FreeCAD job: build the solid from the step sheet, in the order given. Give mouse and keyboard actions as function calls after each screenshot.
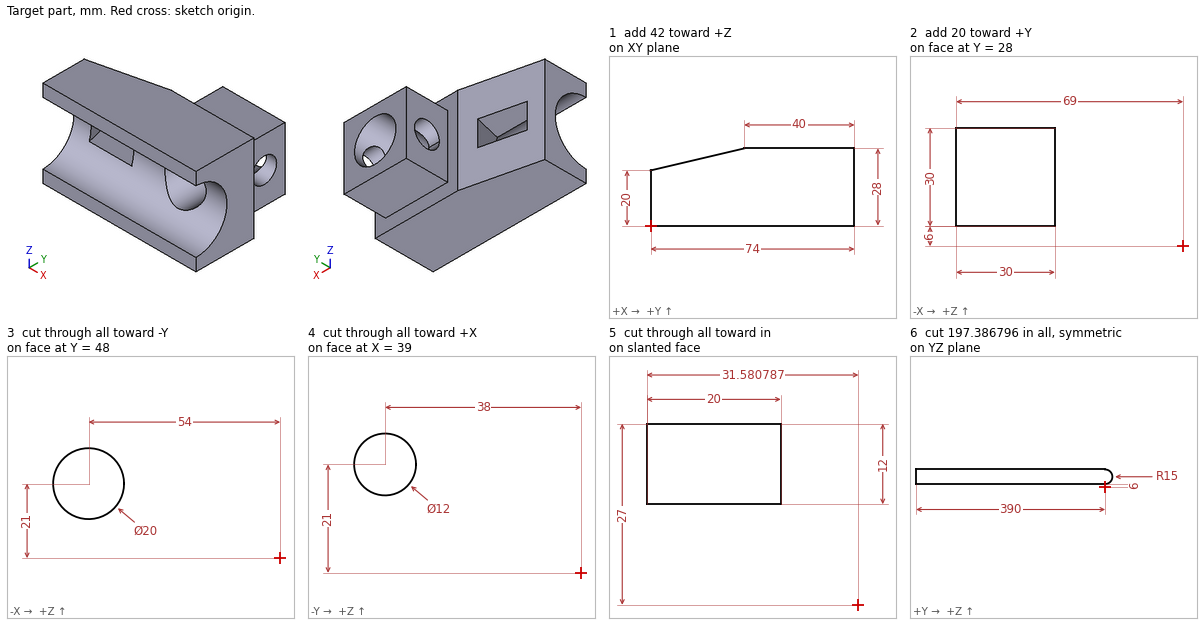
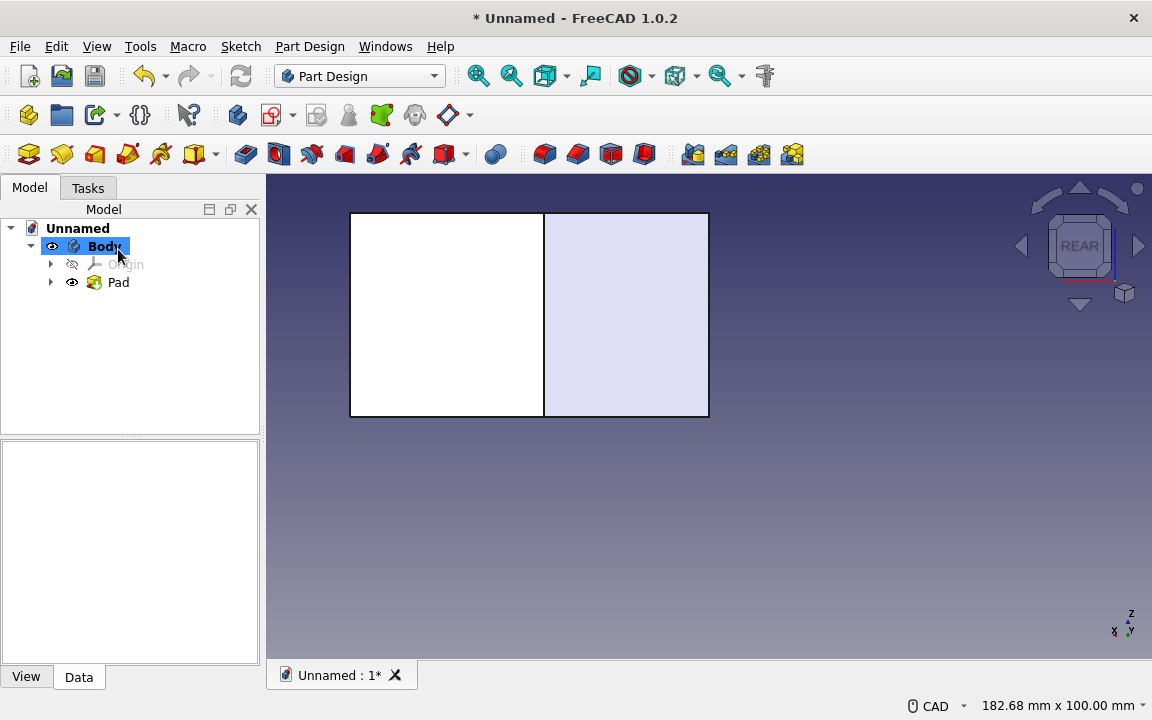
click(479, 76)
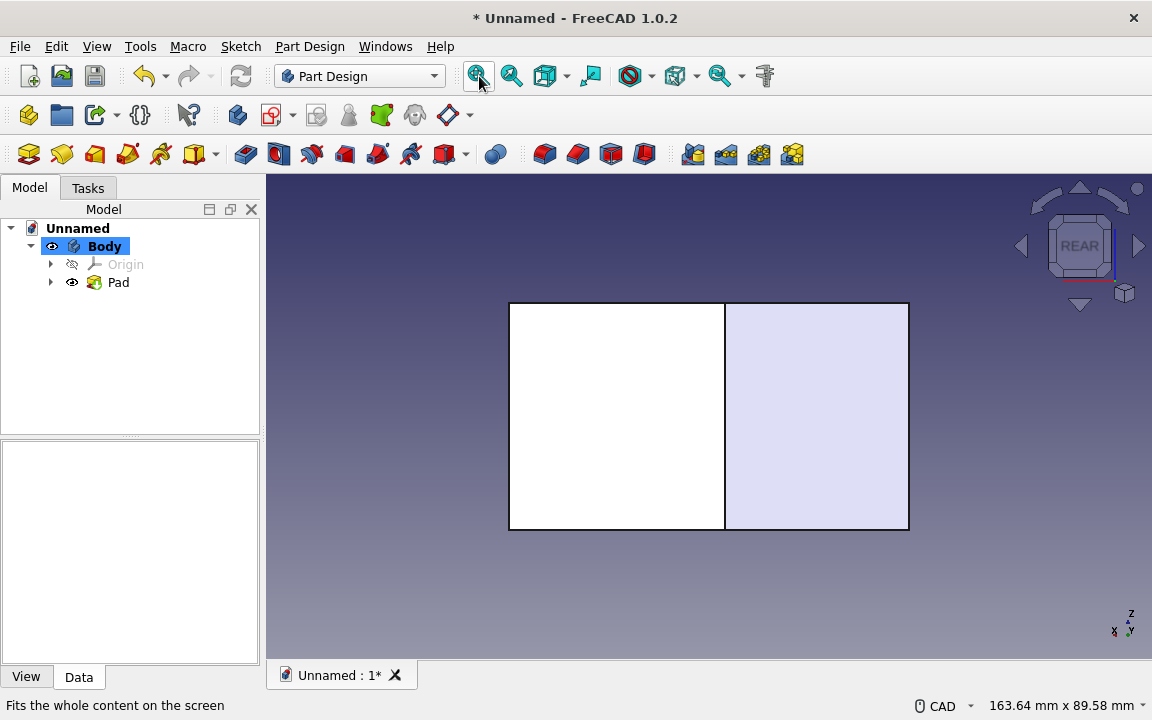
click(617, 416)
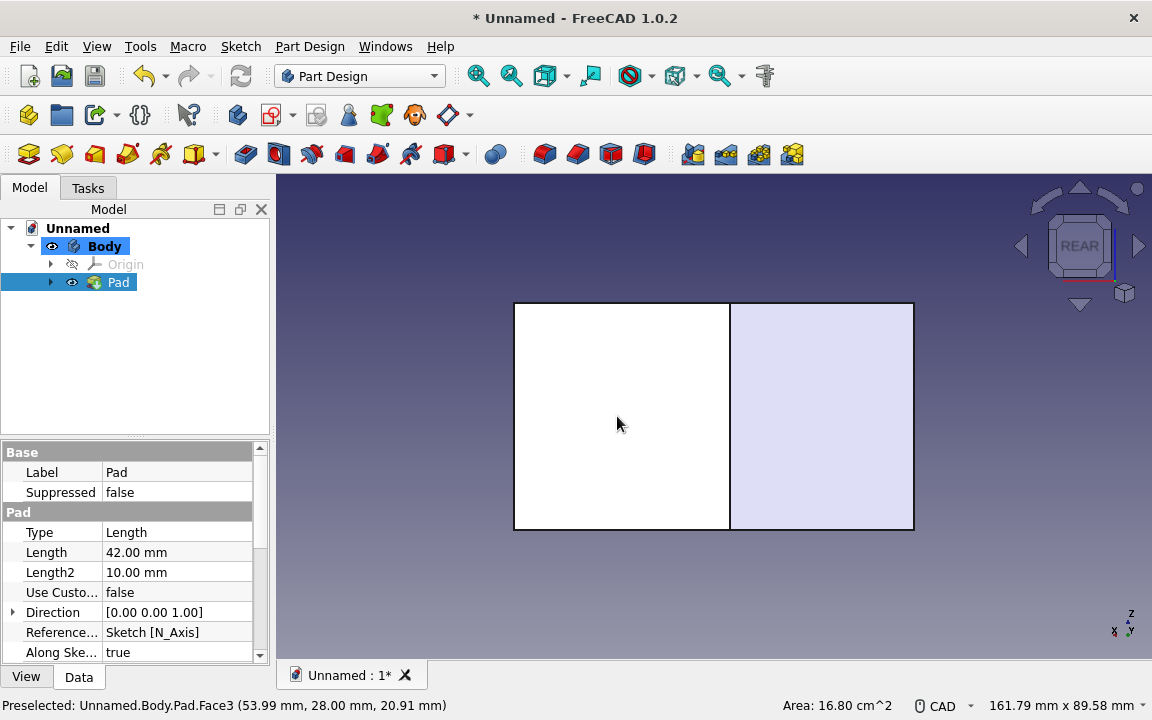
click(270, 116)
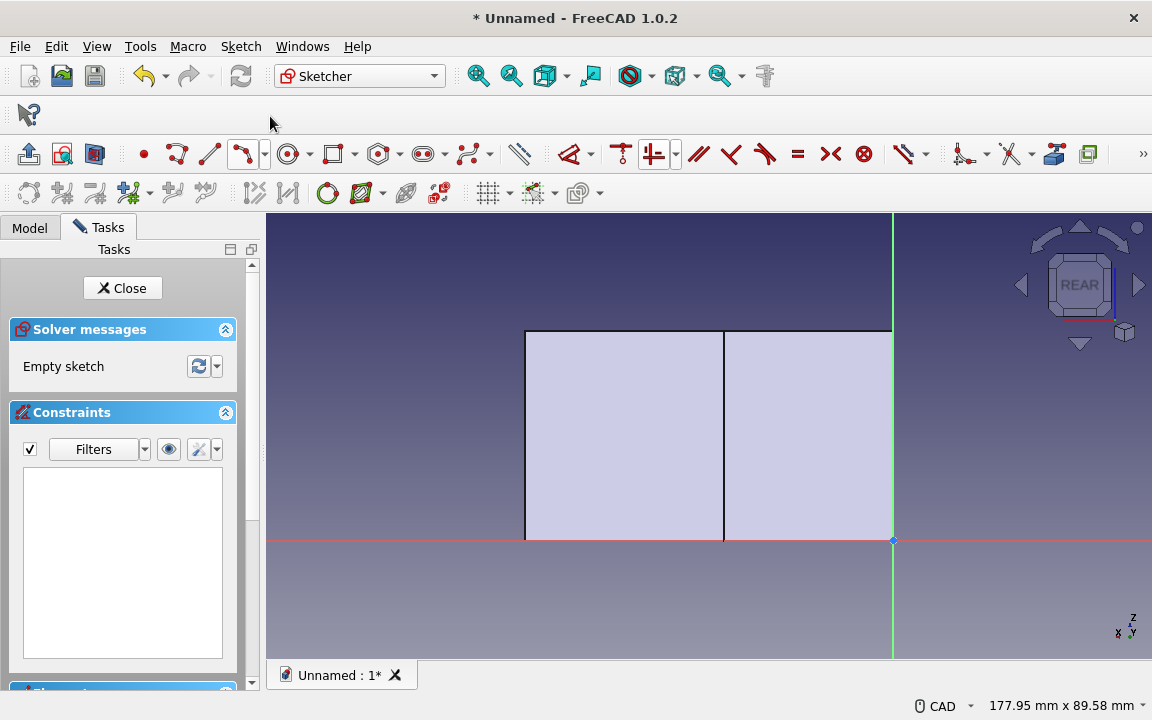
scroll(886, 481, up, 2)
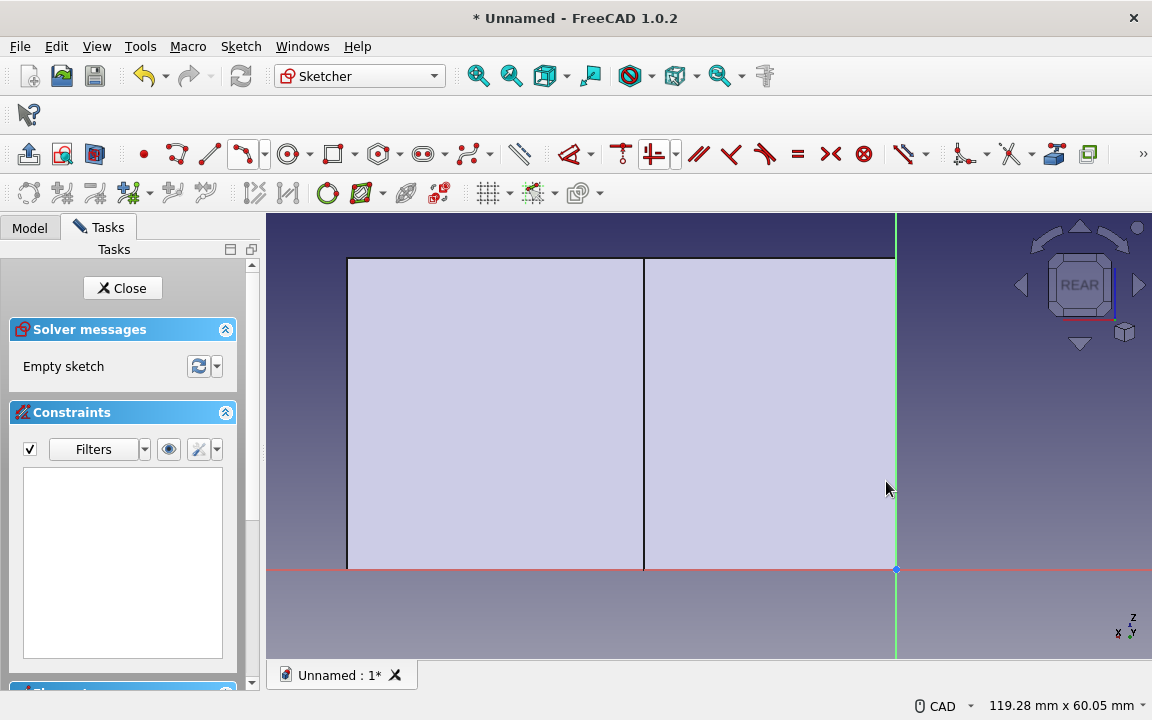
click(332, 154)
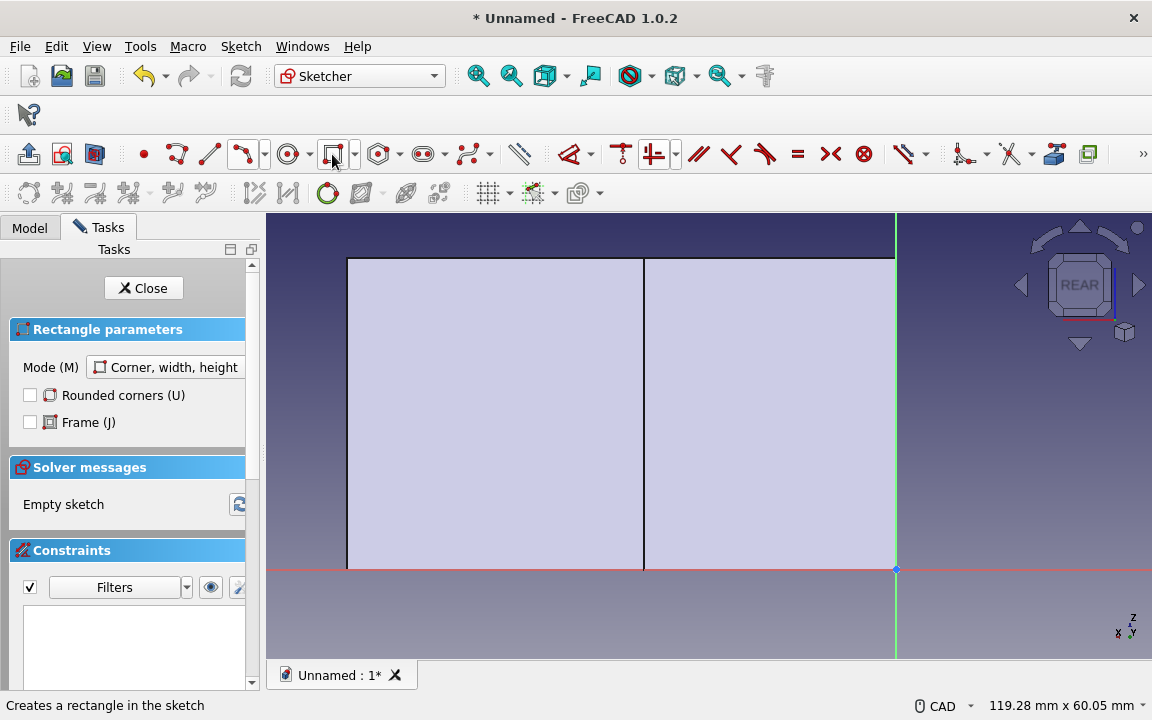
click(384, 302)
move(607, 525)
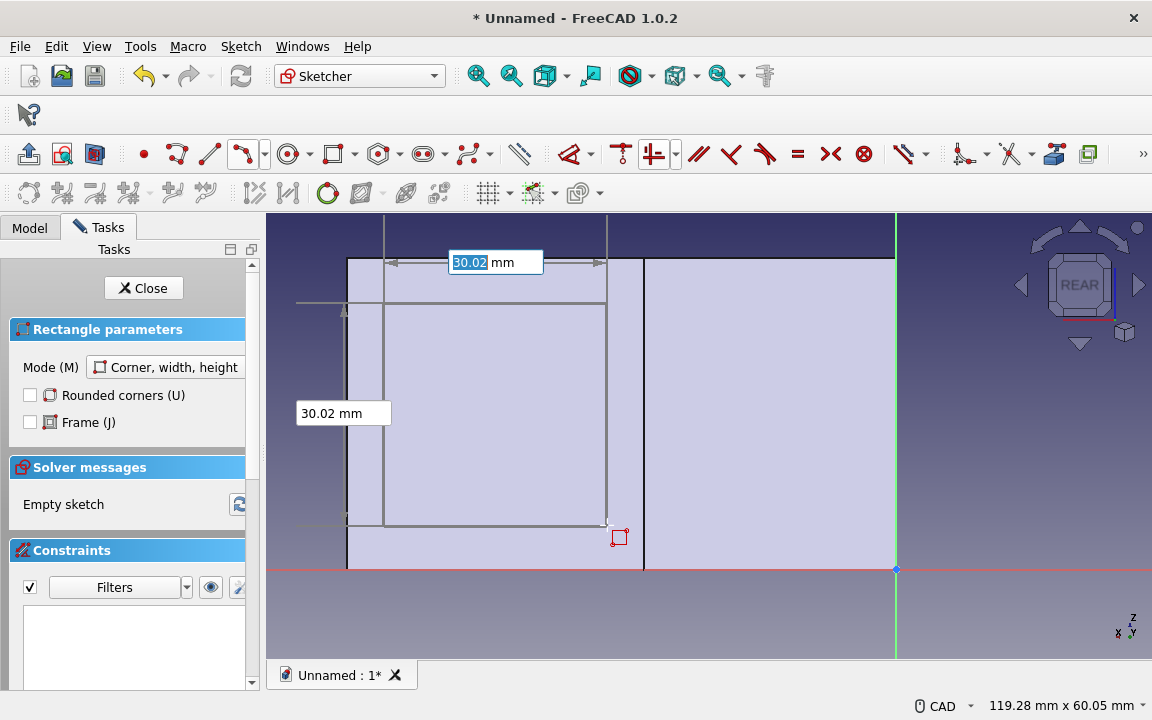
text(30)
key(Tab)
text(30)
key(Return)
key(Escape)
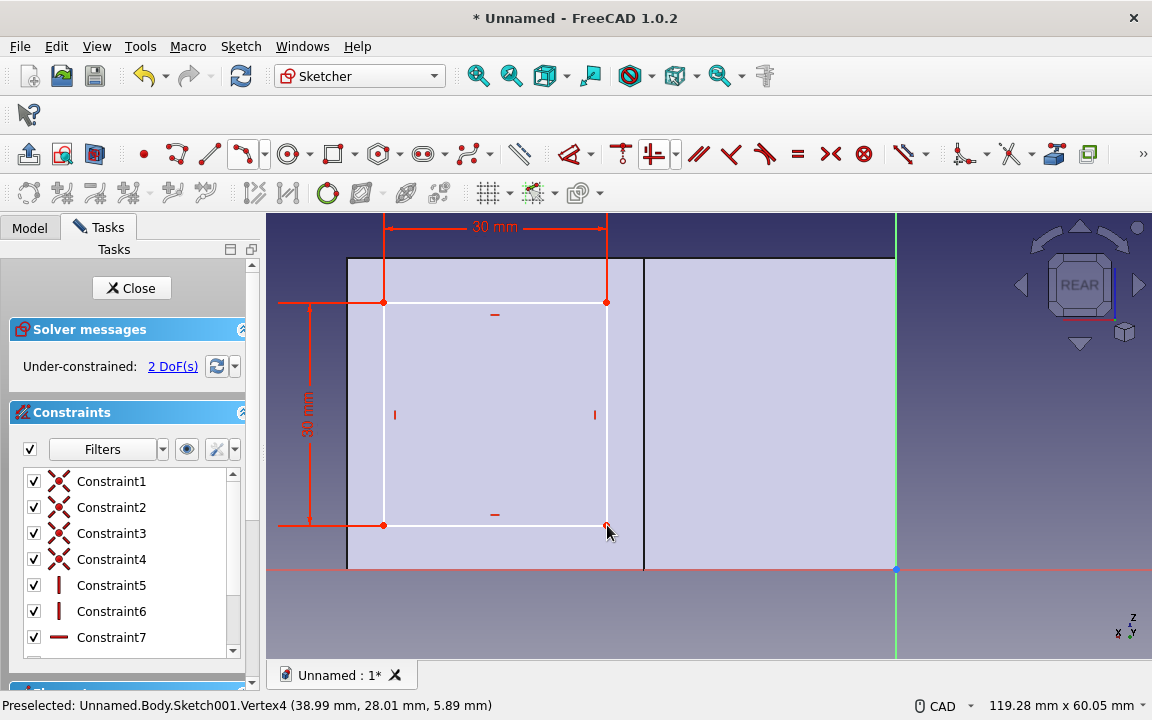
click(568, 154)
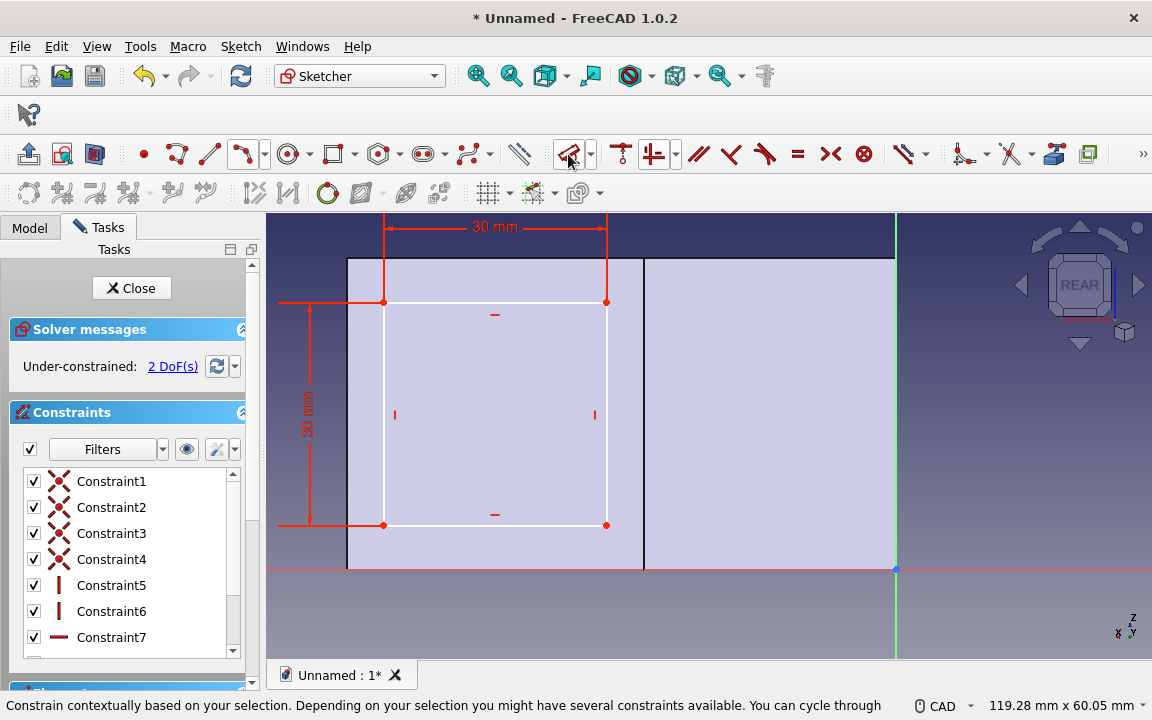
click(384, 526)
click(930, 548)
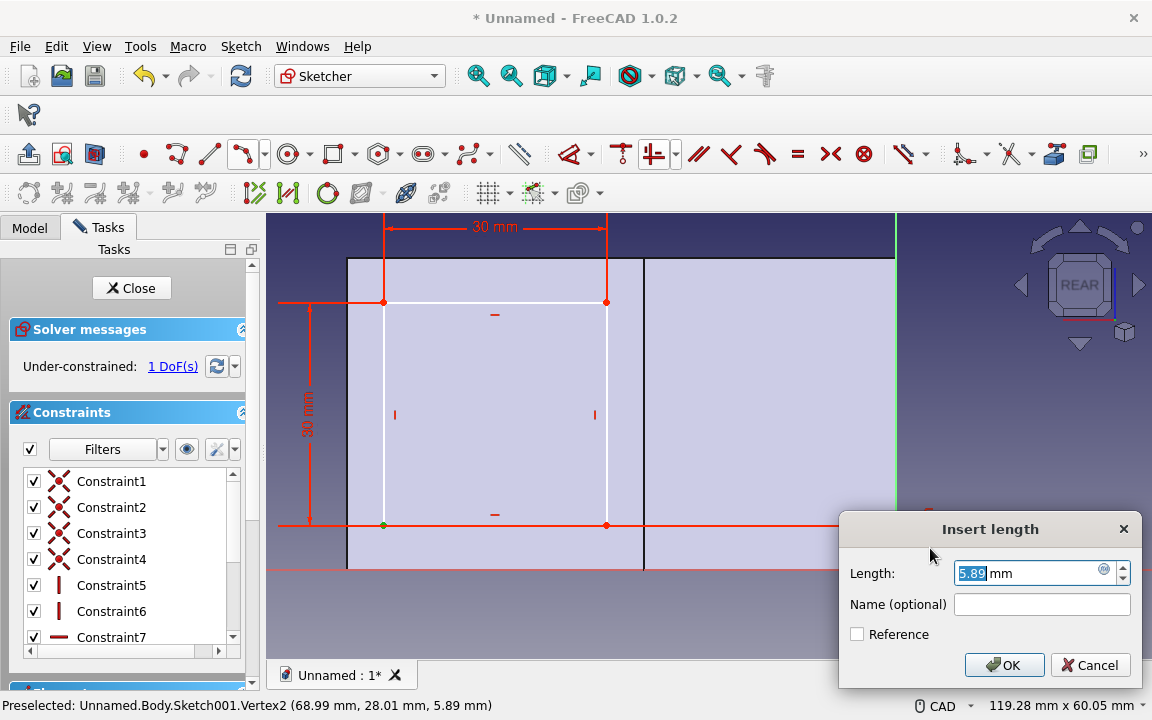
text(6)
key(Return)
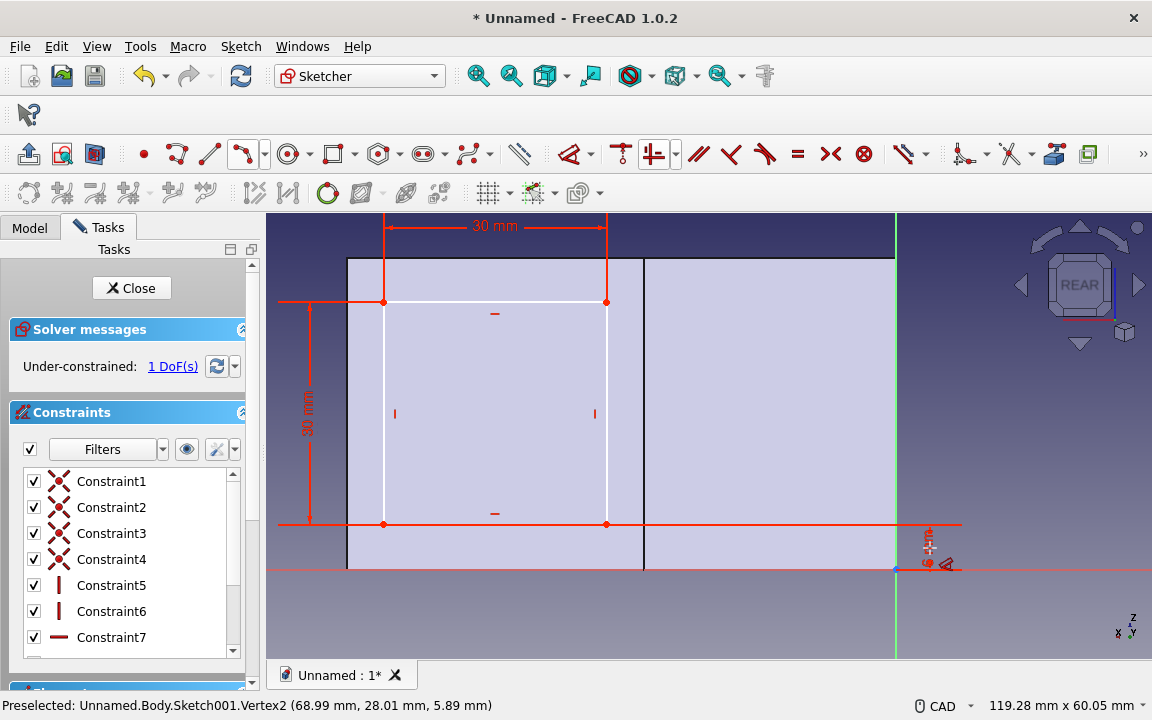
click(384, 302)
click(640, 604)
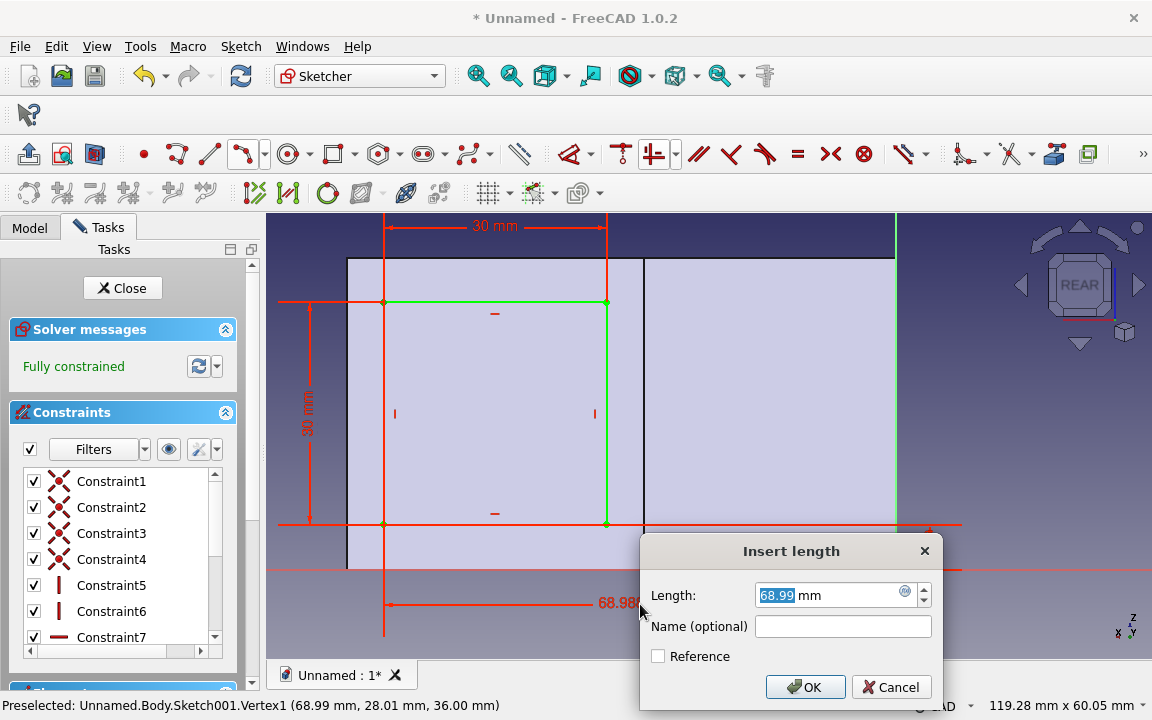
text(69)
key(Return)
key(Escape)